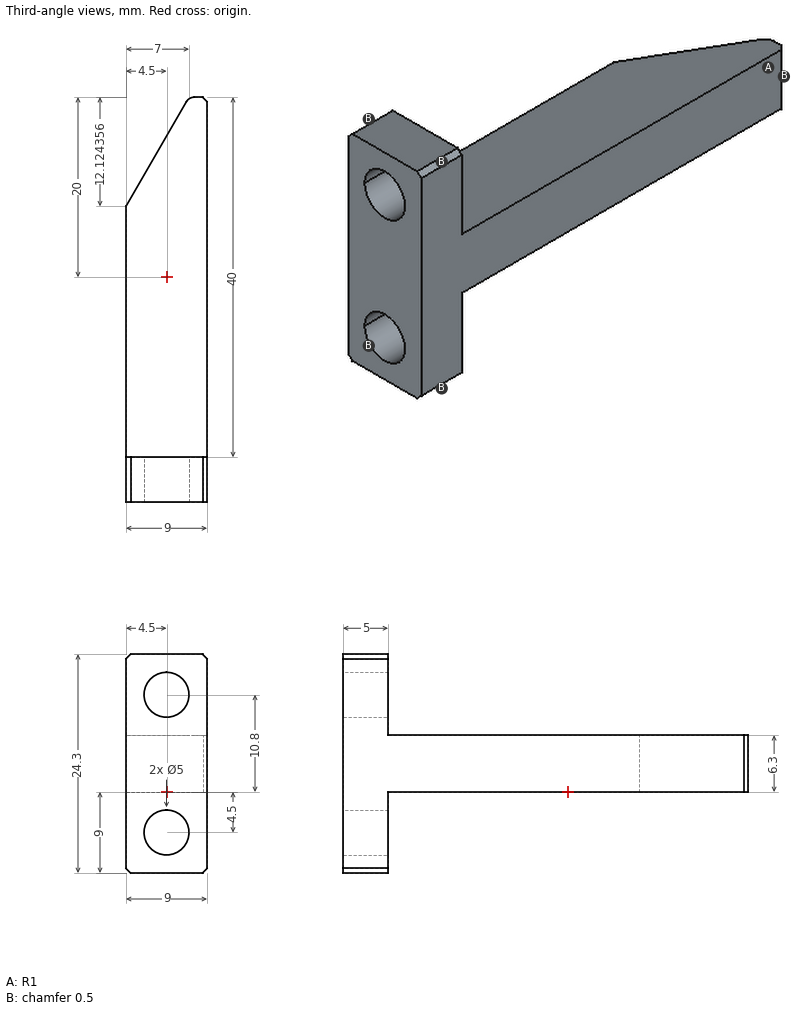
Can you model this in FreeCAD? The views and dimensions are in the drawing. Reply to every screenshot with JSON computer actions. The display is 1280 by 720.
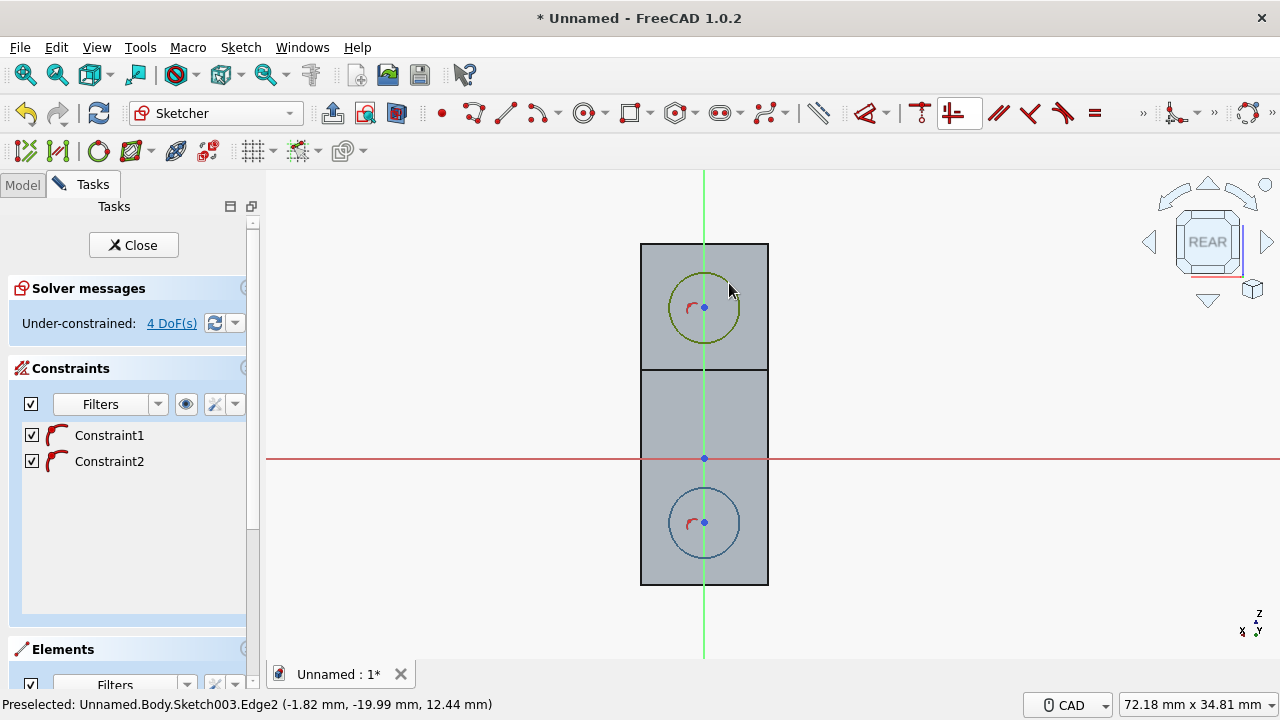
{"action": "left_click", "coordinate": [1096, 114]}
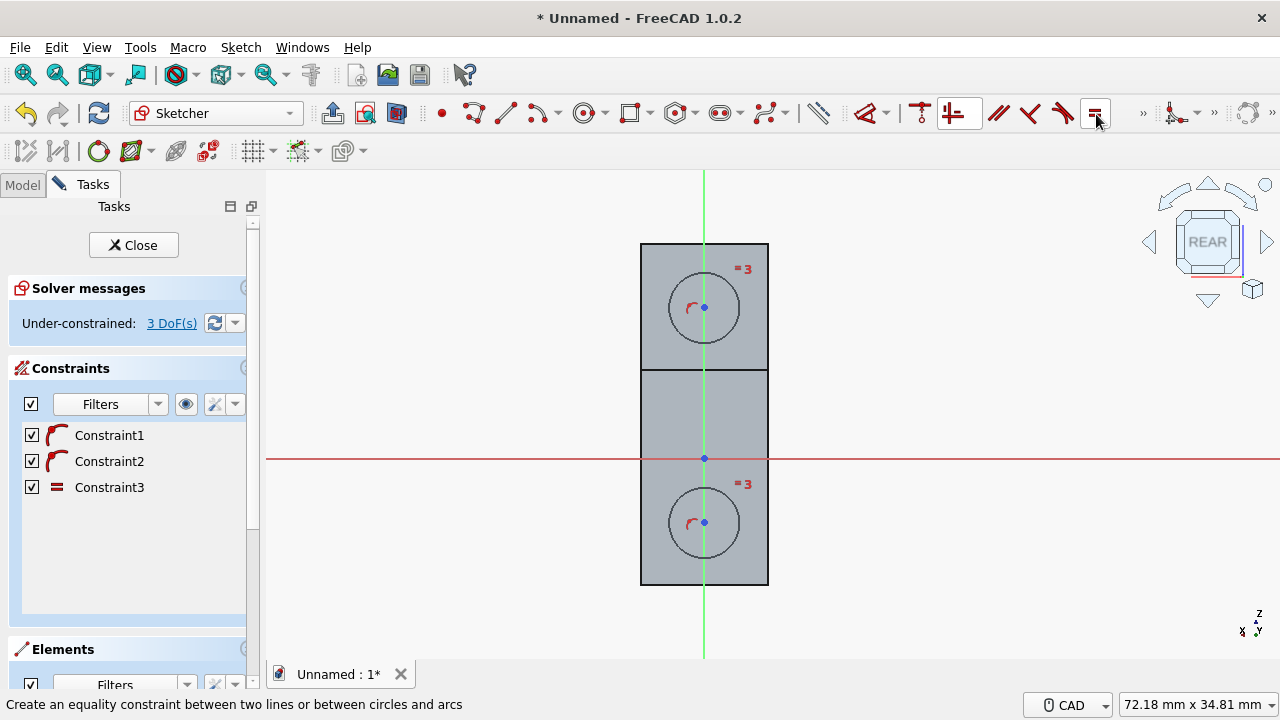
{"action": "left_click", "coordinate": [866, 114]}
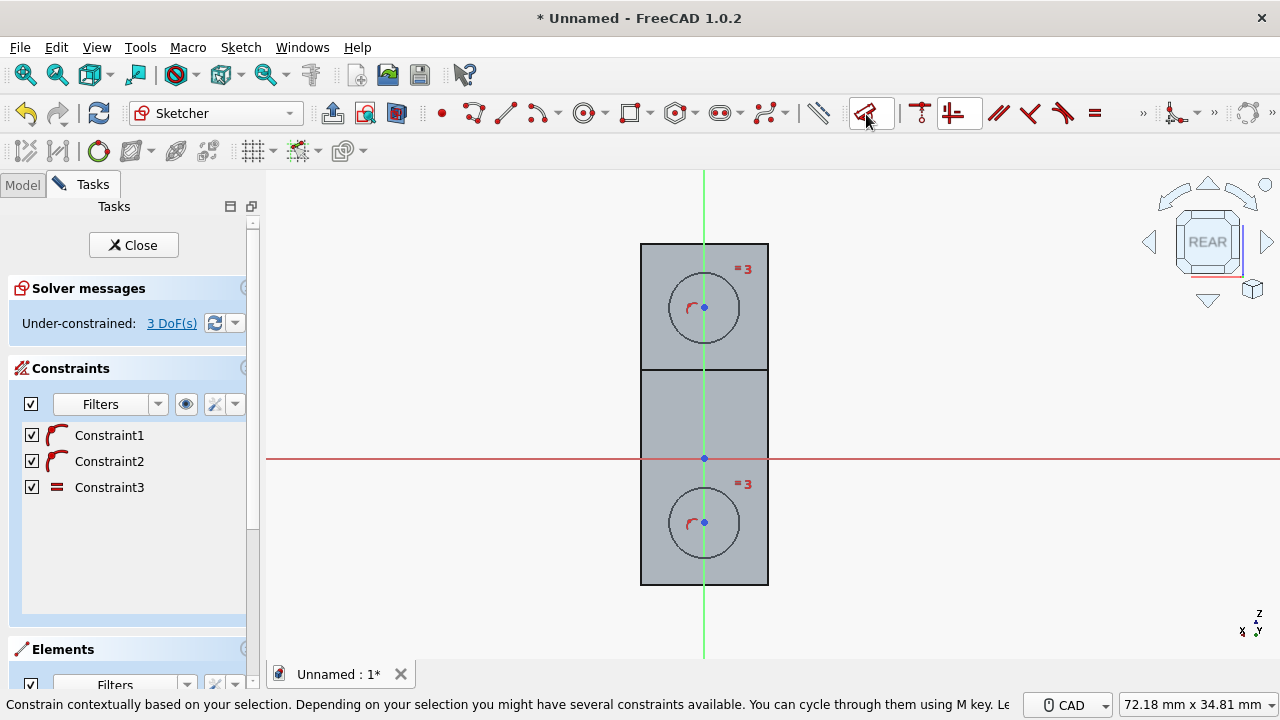
{"action": "left_click", "coordinate": [729, 498]}
{"action": "left_click", "coordinate": [751, 475]}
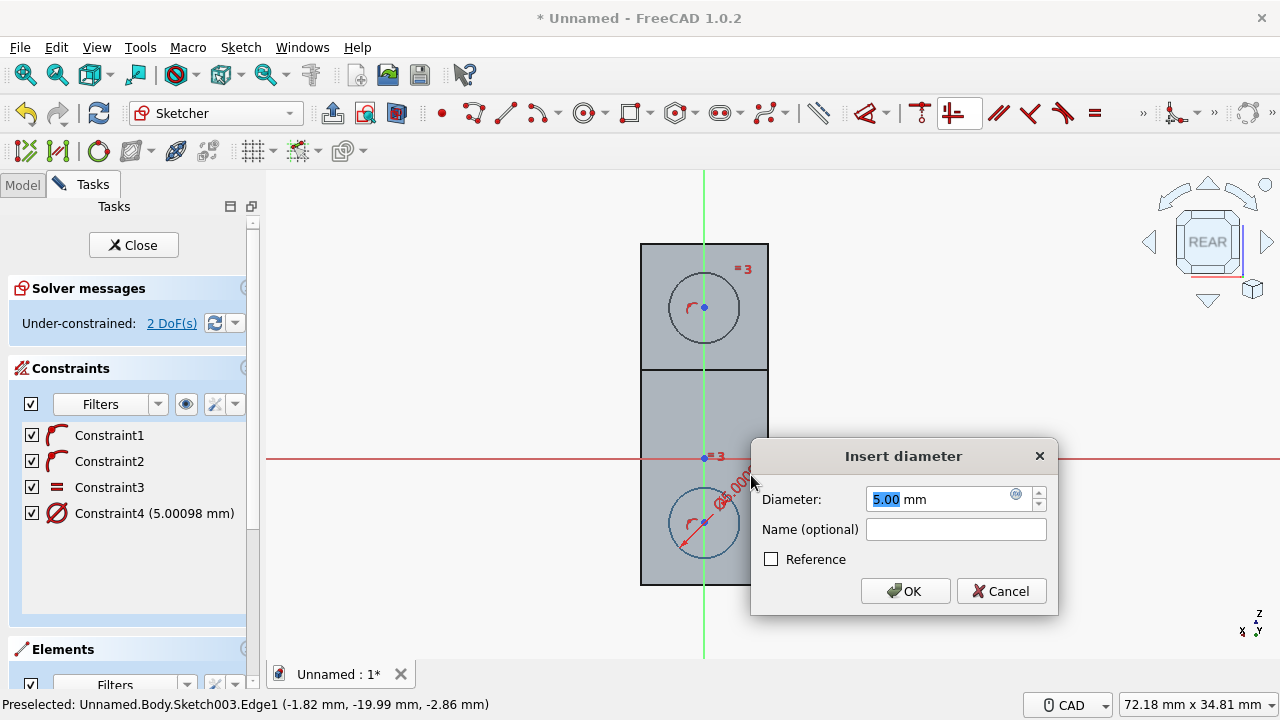
{"action": "type", "text": "5"}
{"action": "key", "text": "Return"}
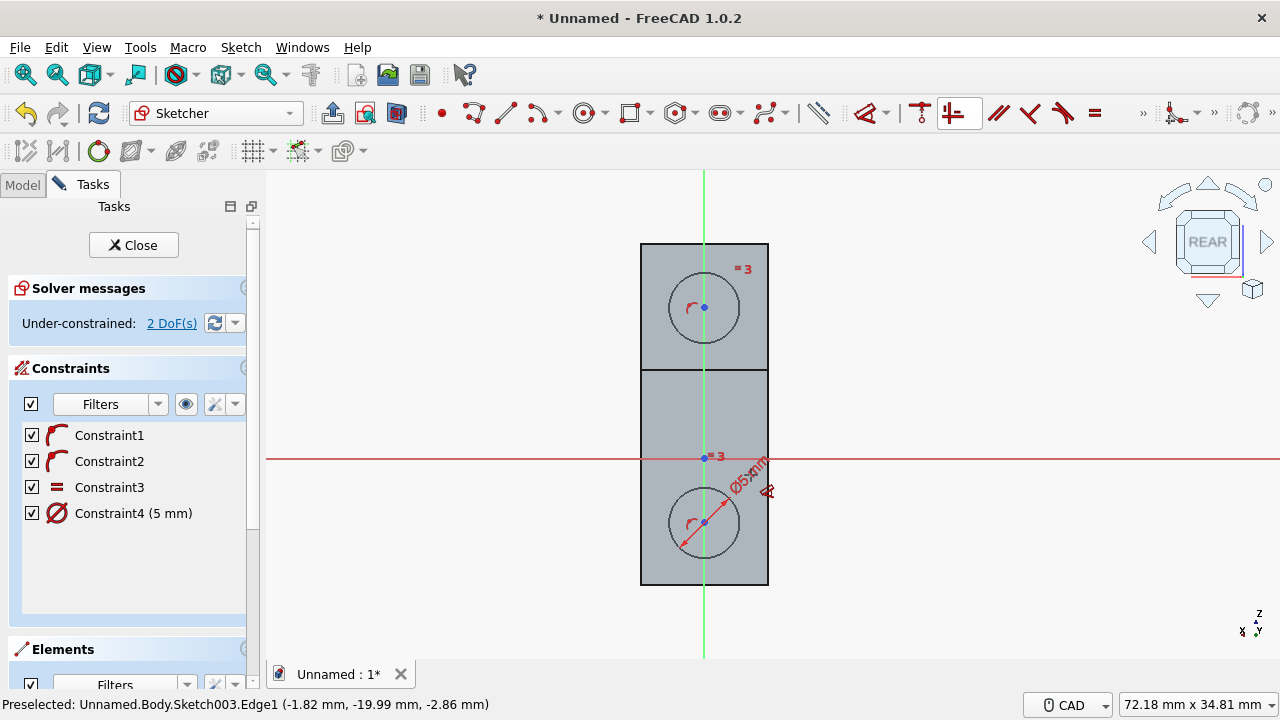
{"action": "left_click", "coordinate": [704, 523]}
{"action": "left_click", "coordinate": [670, 476]}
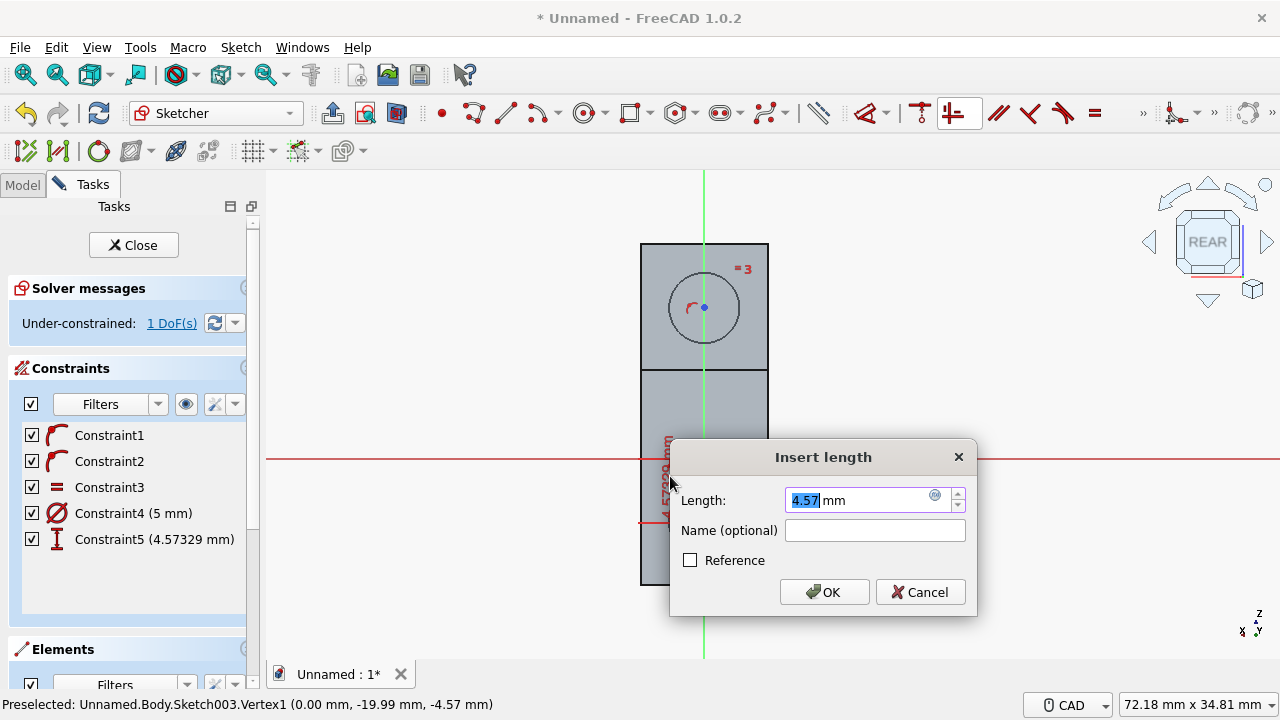
{"action": "type", "text": "4.5"}
{"action": "key", "text": "Return"}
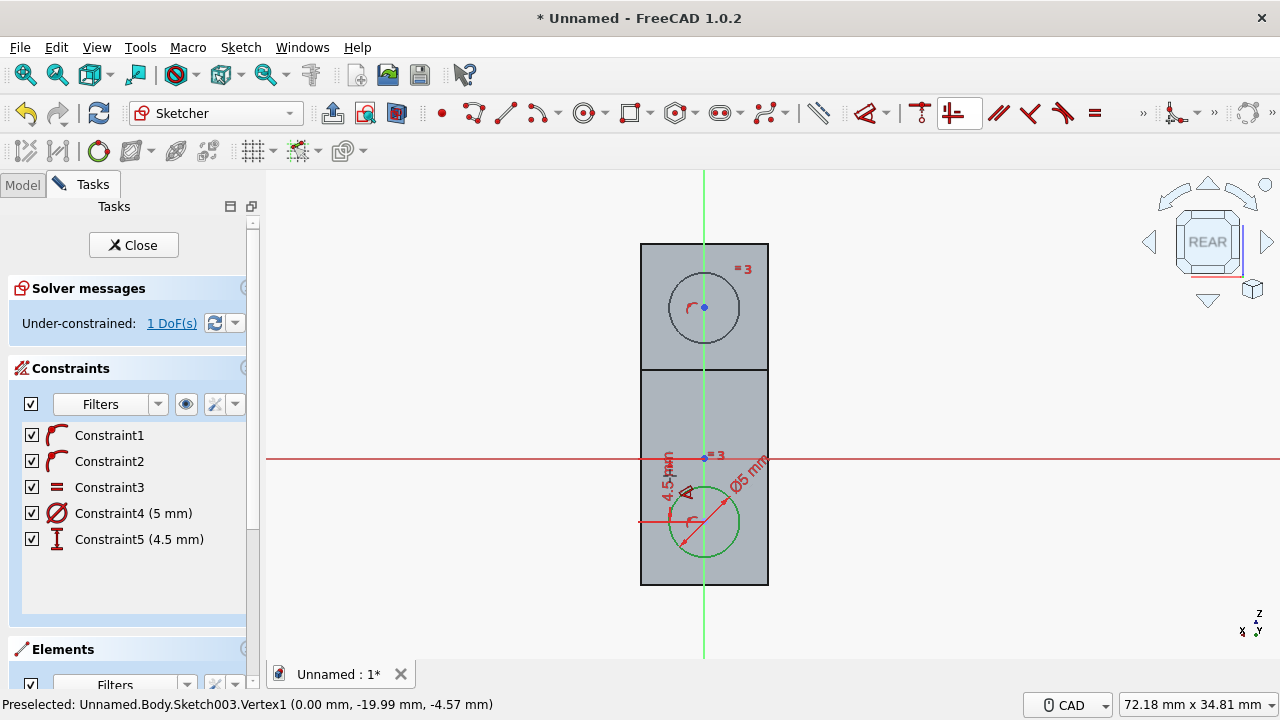
{"action": "left_click", "coordinate": [704, 308]}
{"action": "left_click", "coordinate": [738, 383]}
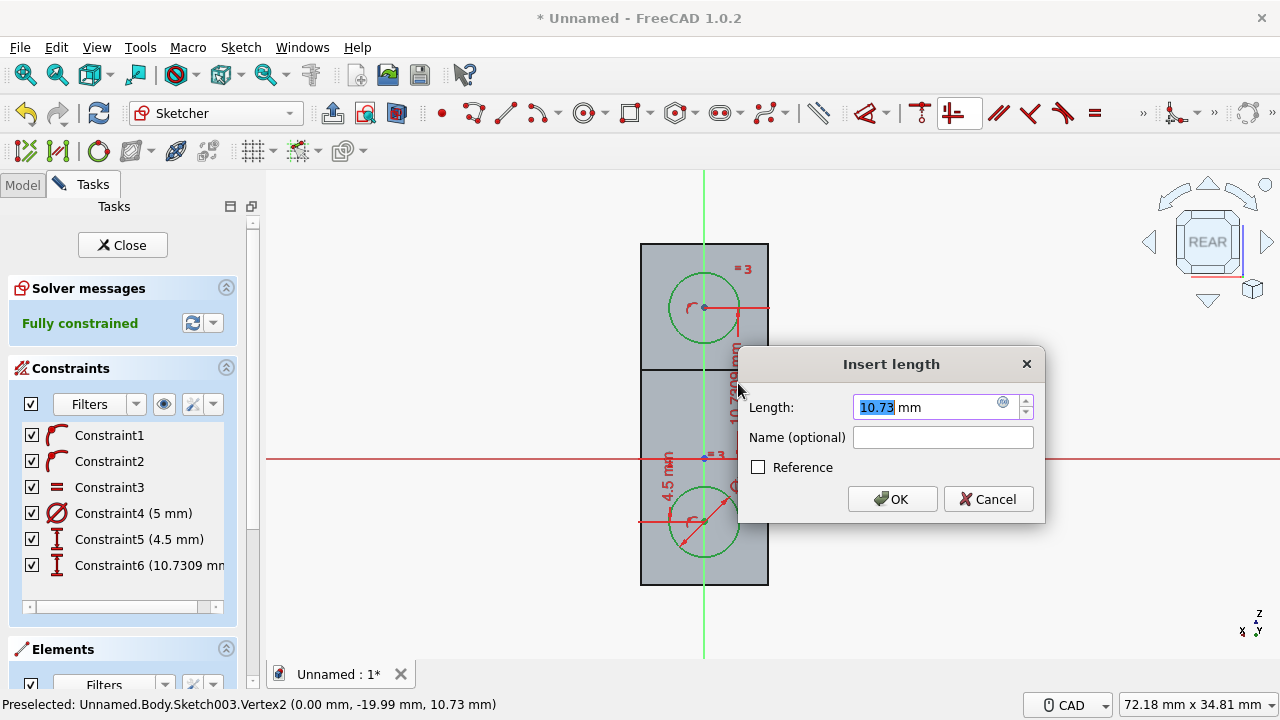
{"action": "type", "text": "10.8"}
{"action": "key", "text": "Return"}
{"action": "key", "text": "Escape"}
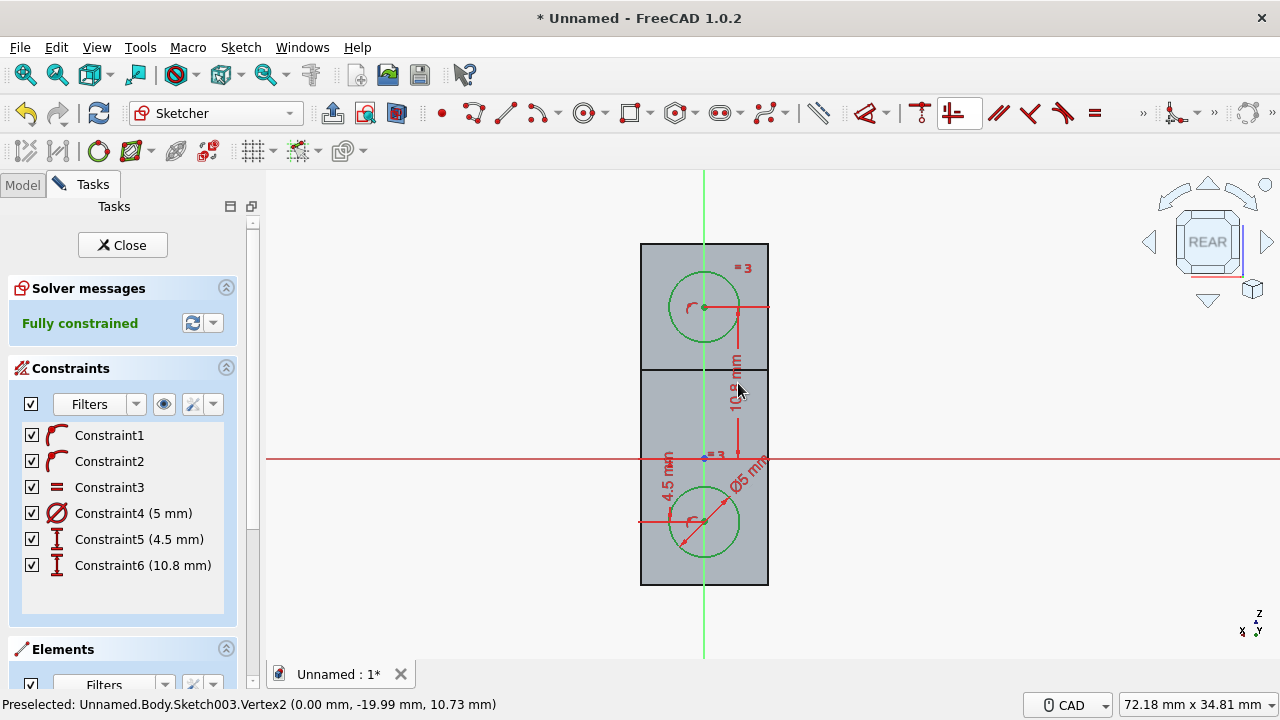
{"action": "left_click", "coordinate": [123, 245]}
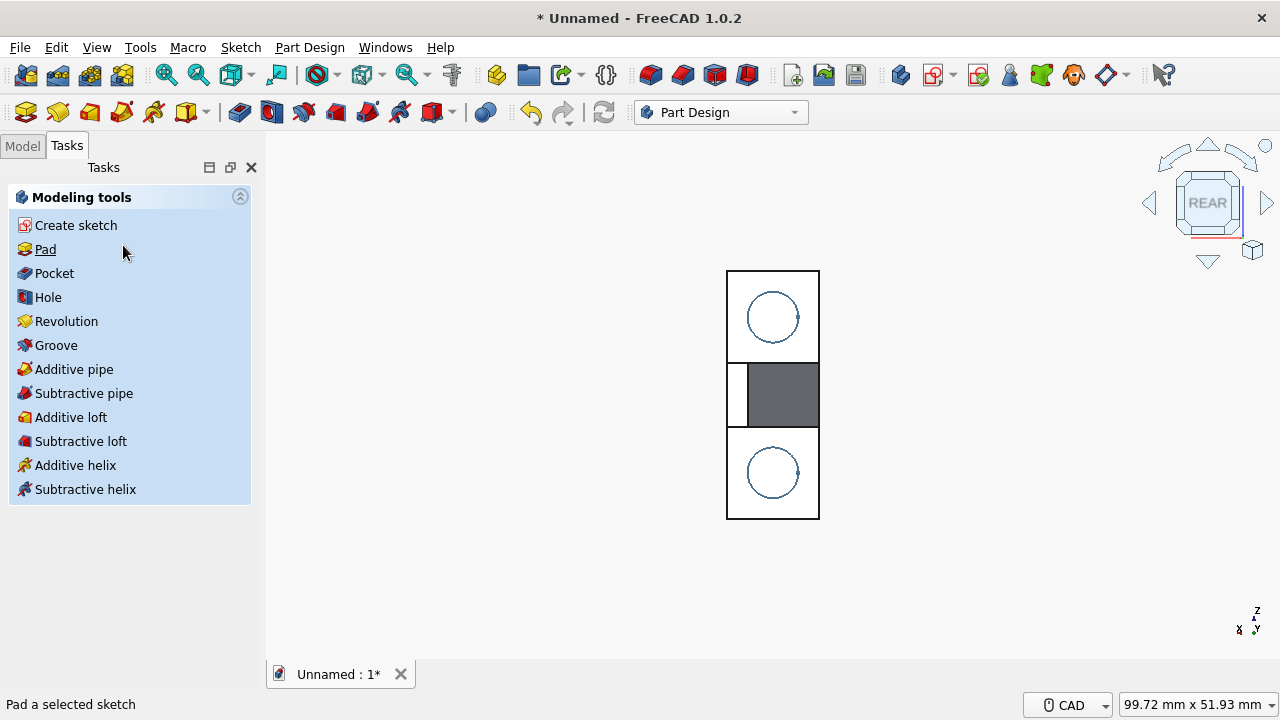
{"action": "left_click", "coordinate": [240, 112]}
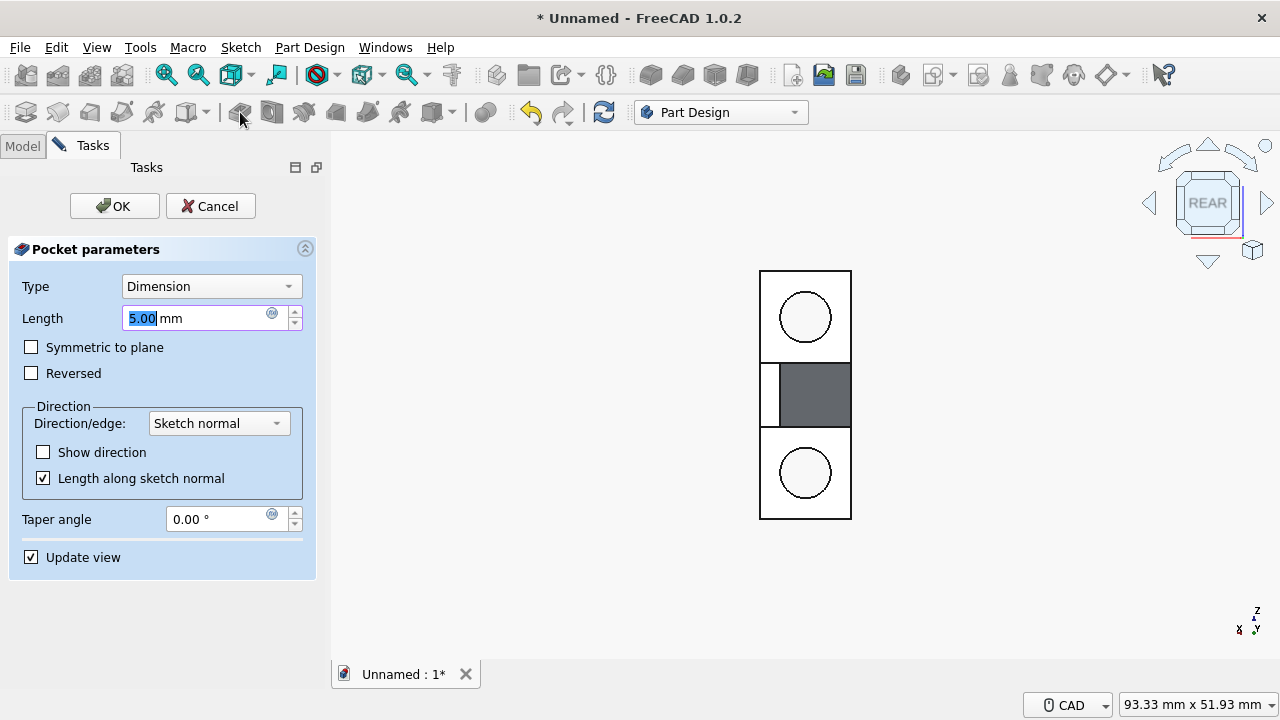
{"action": "left_click", "coordinate": [212, 286]}